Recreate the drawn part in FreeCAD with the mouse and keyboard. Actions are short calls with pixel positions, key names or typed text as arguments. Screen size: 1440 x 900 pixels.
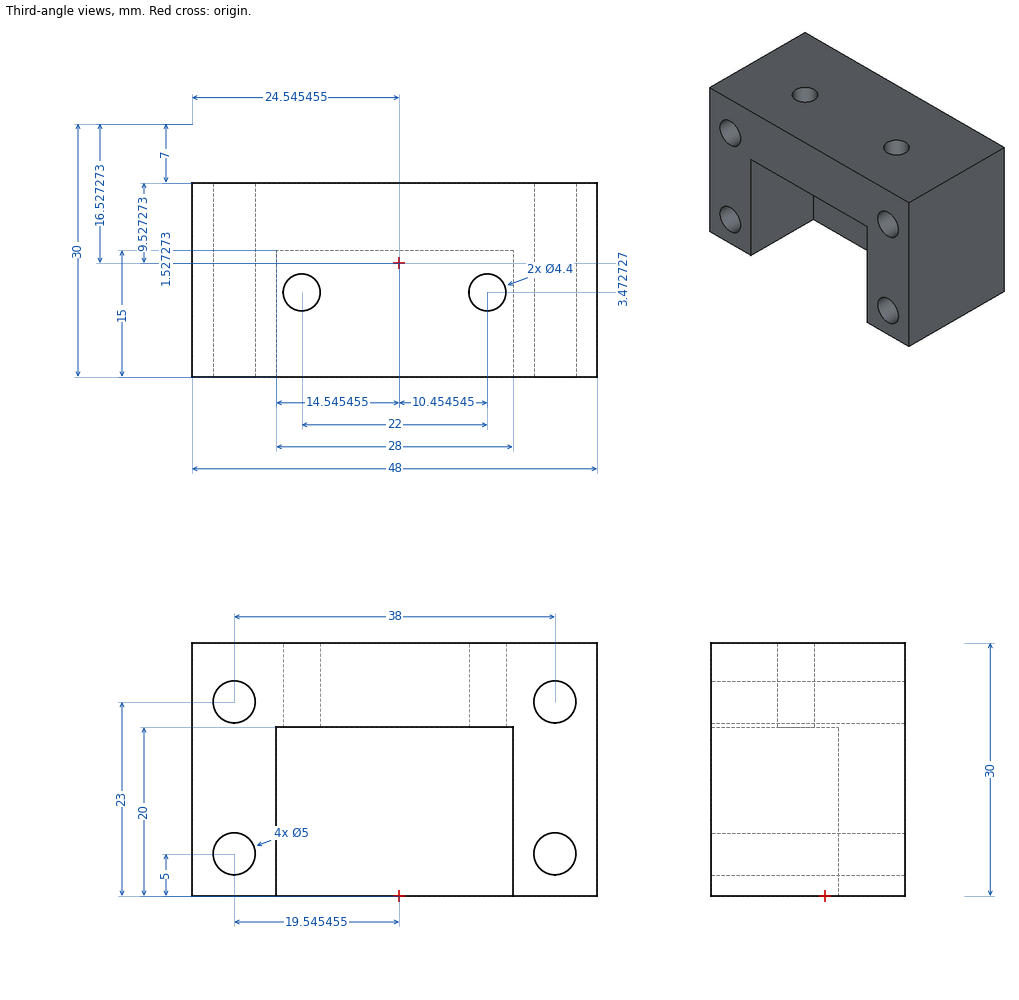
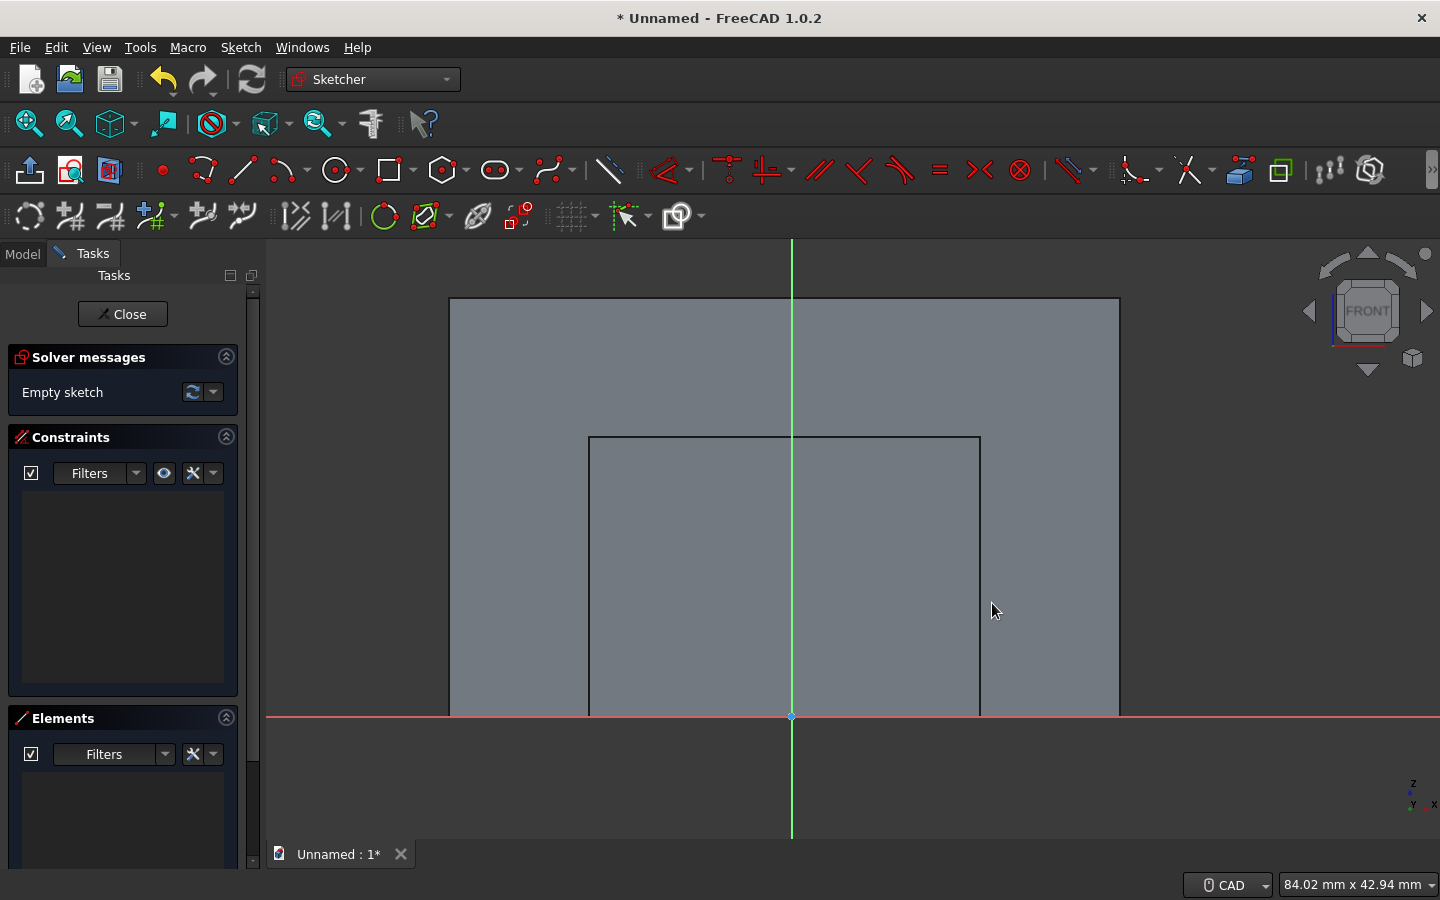
click(336, 170)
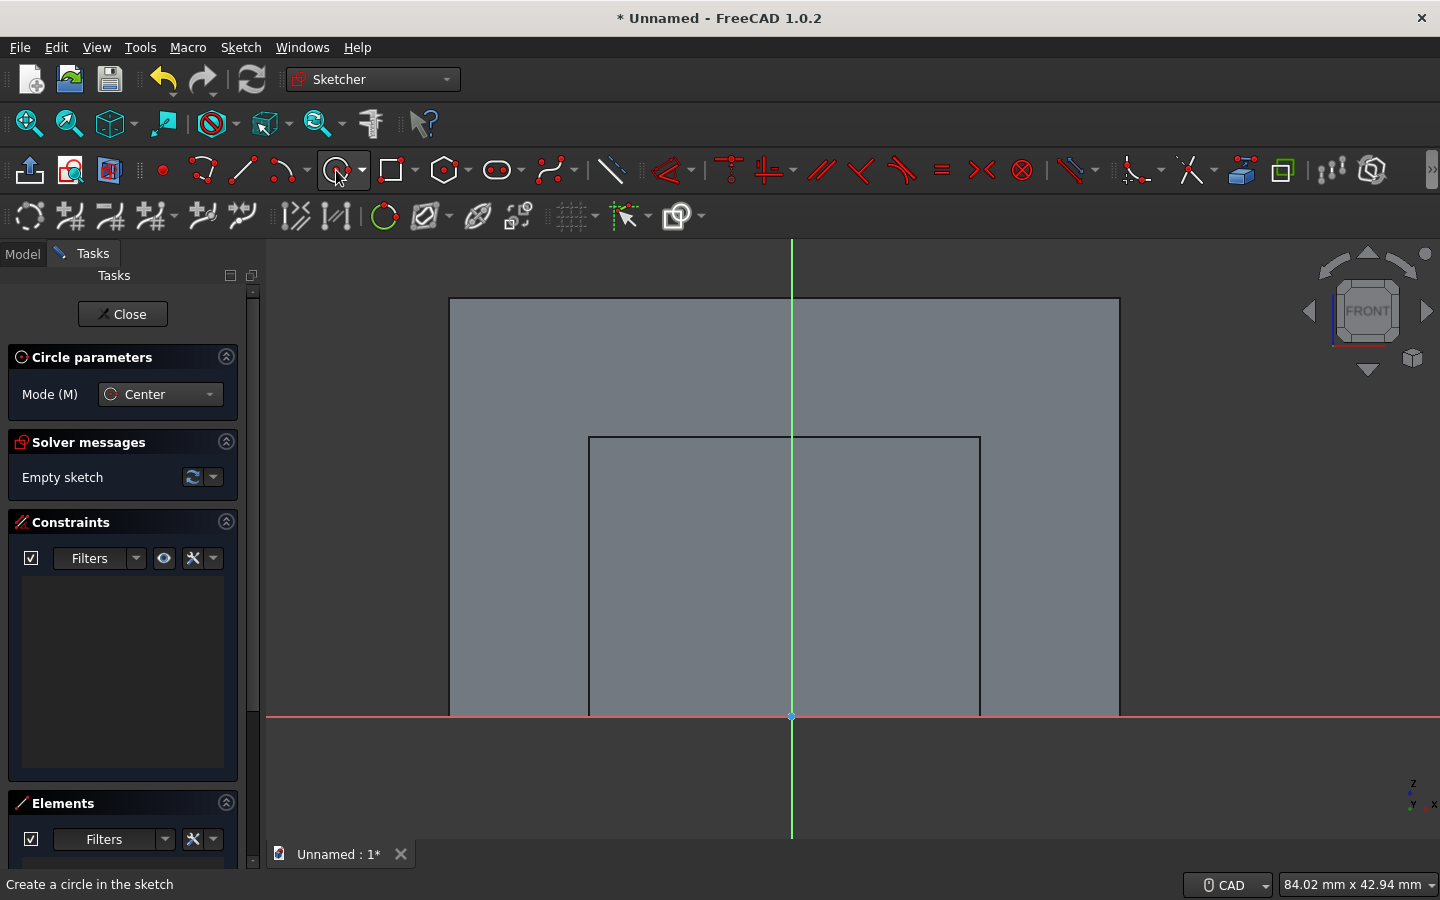
click(519, 647)
click(544, 622)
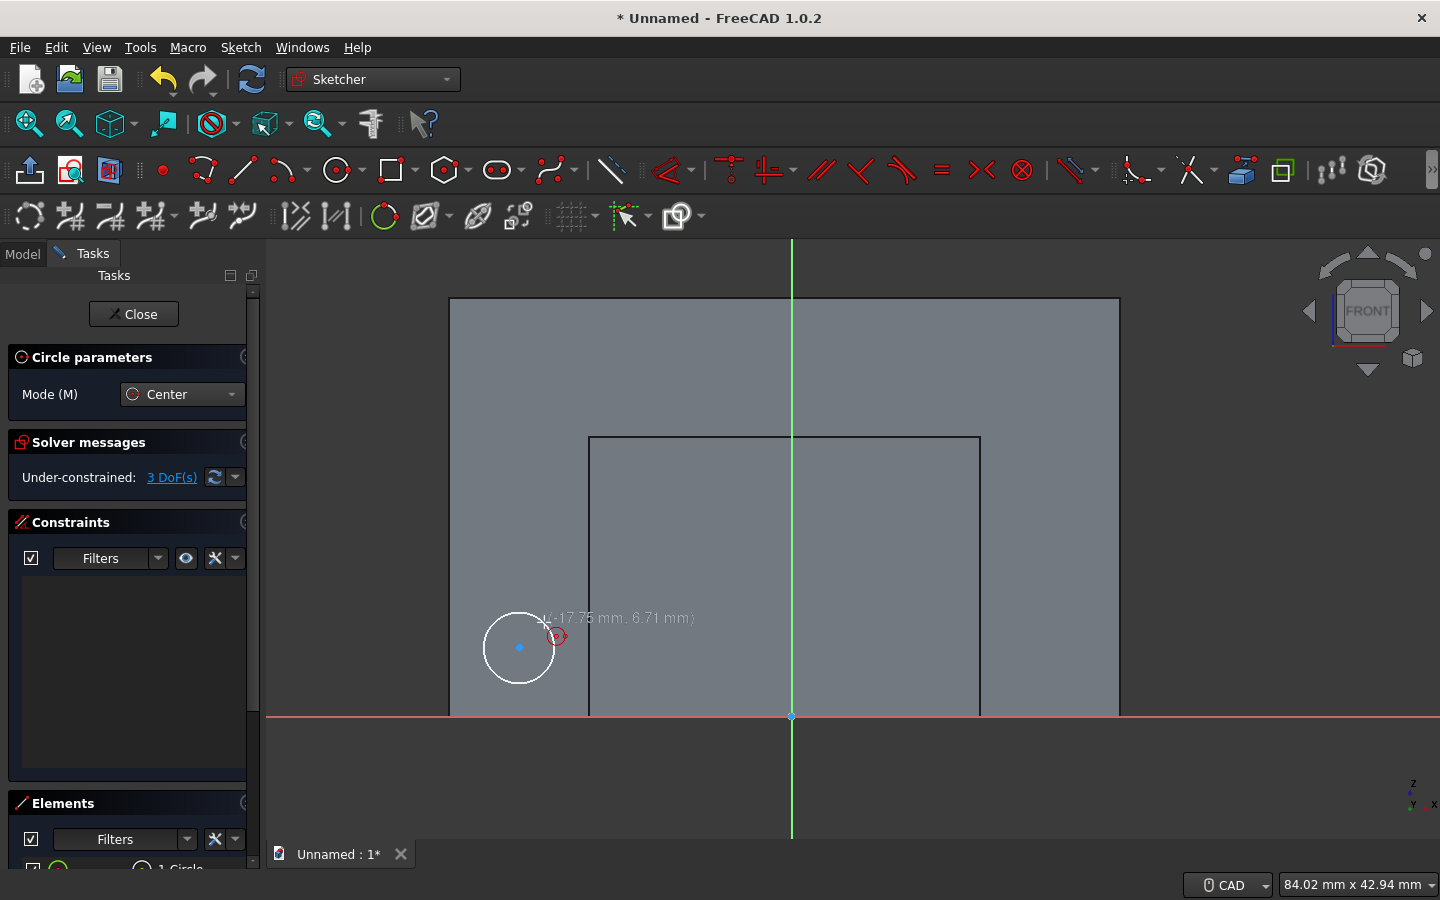
click(519, 395)
click(544, 371)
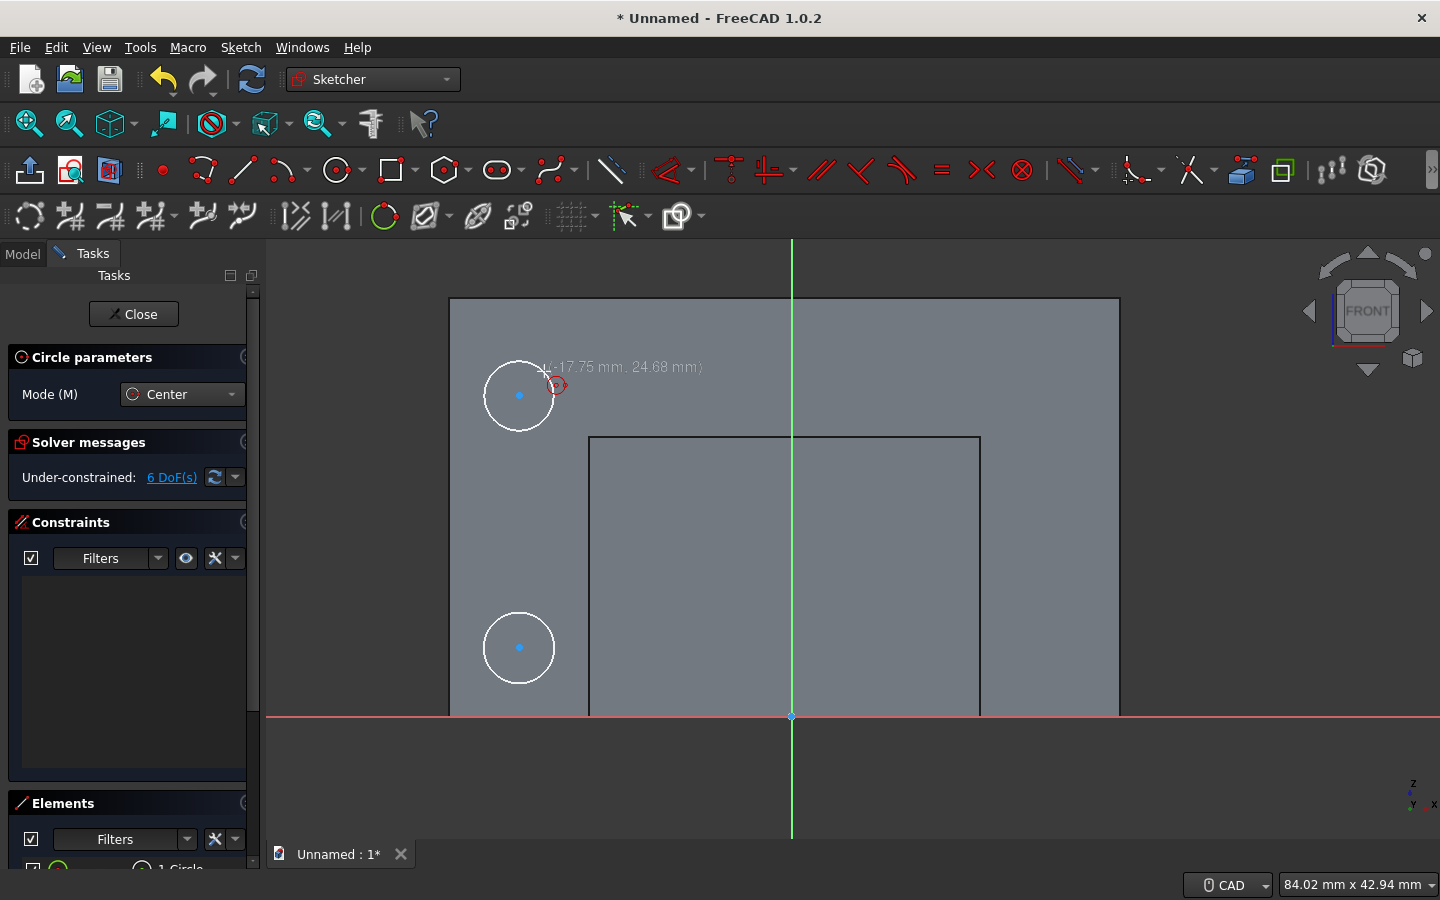
click(1050, 395)
click(1075, 371)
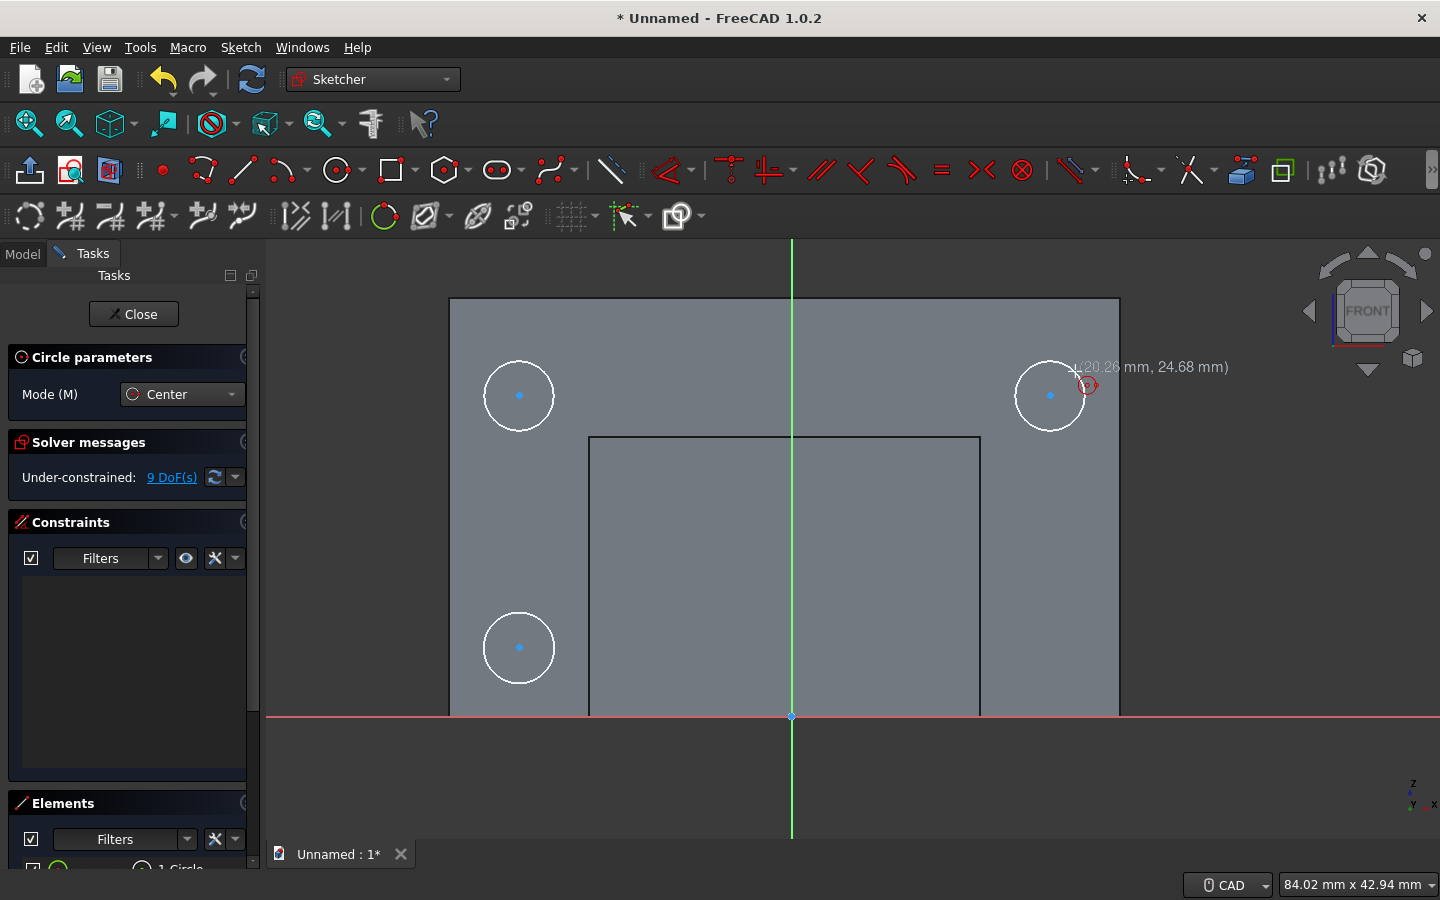
click(1050, 647)
click(1075, 622)
key(Escape)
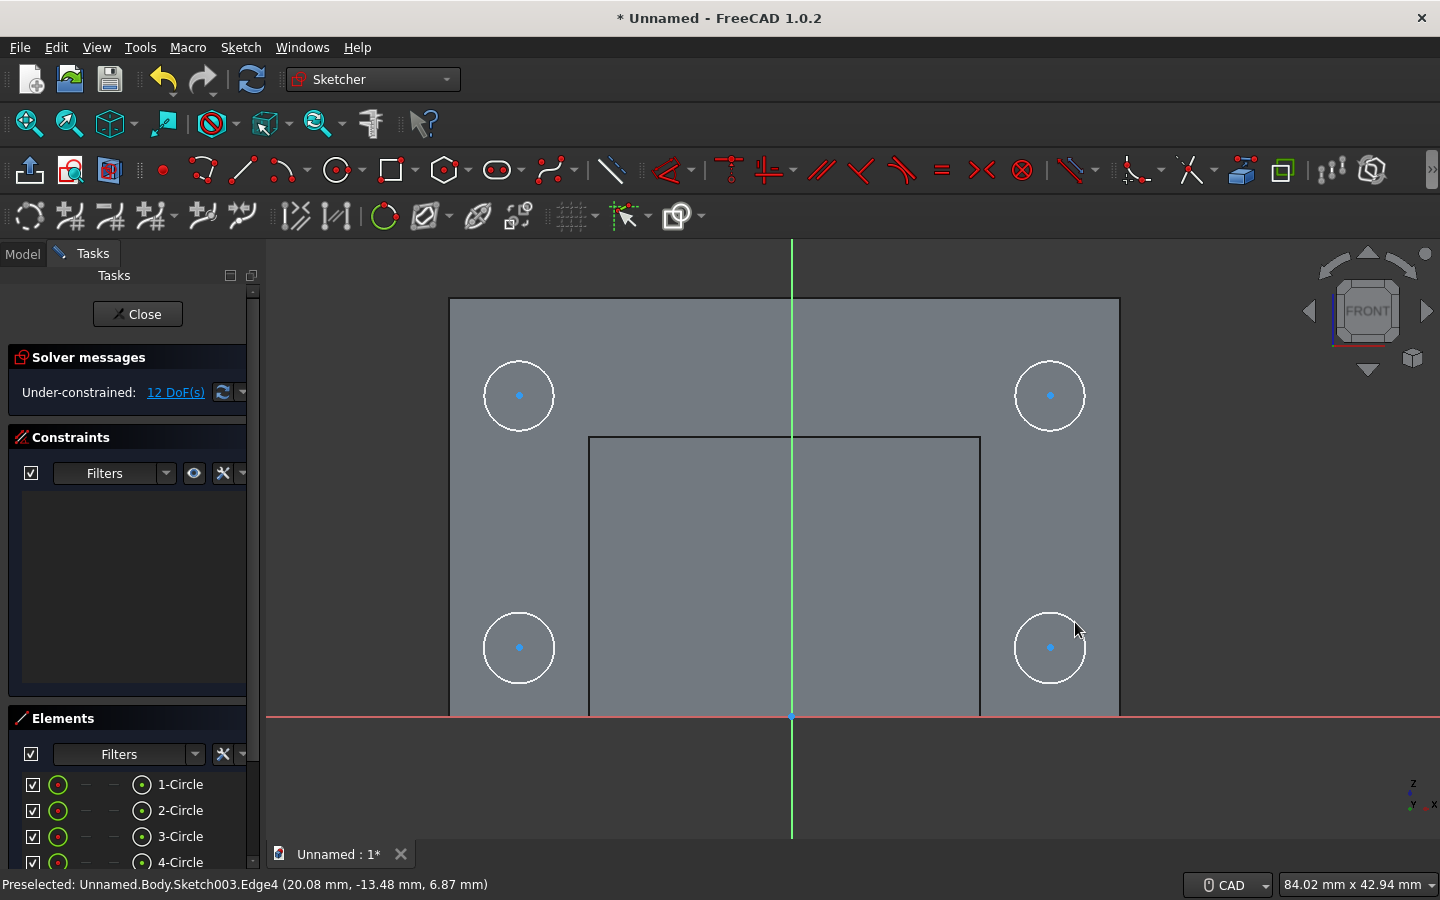
click(544, 623)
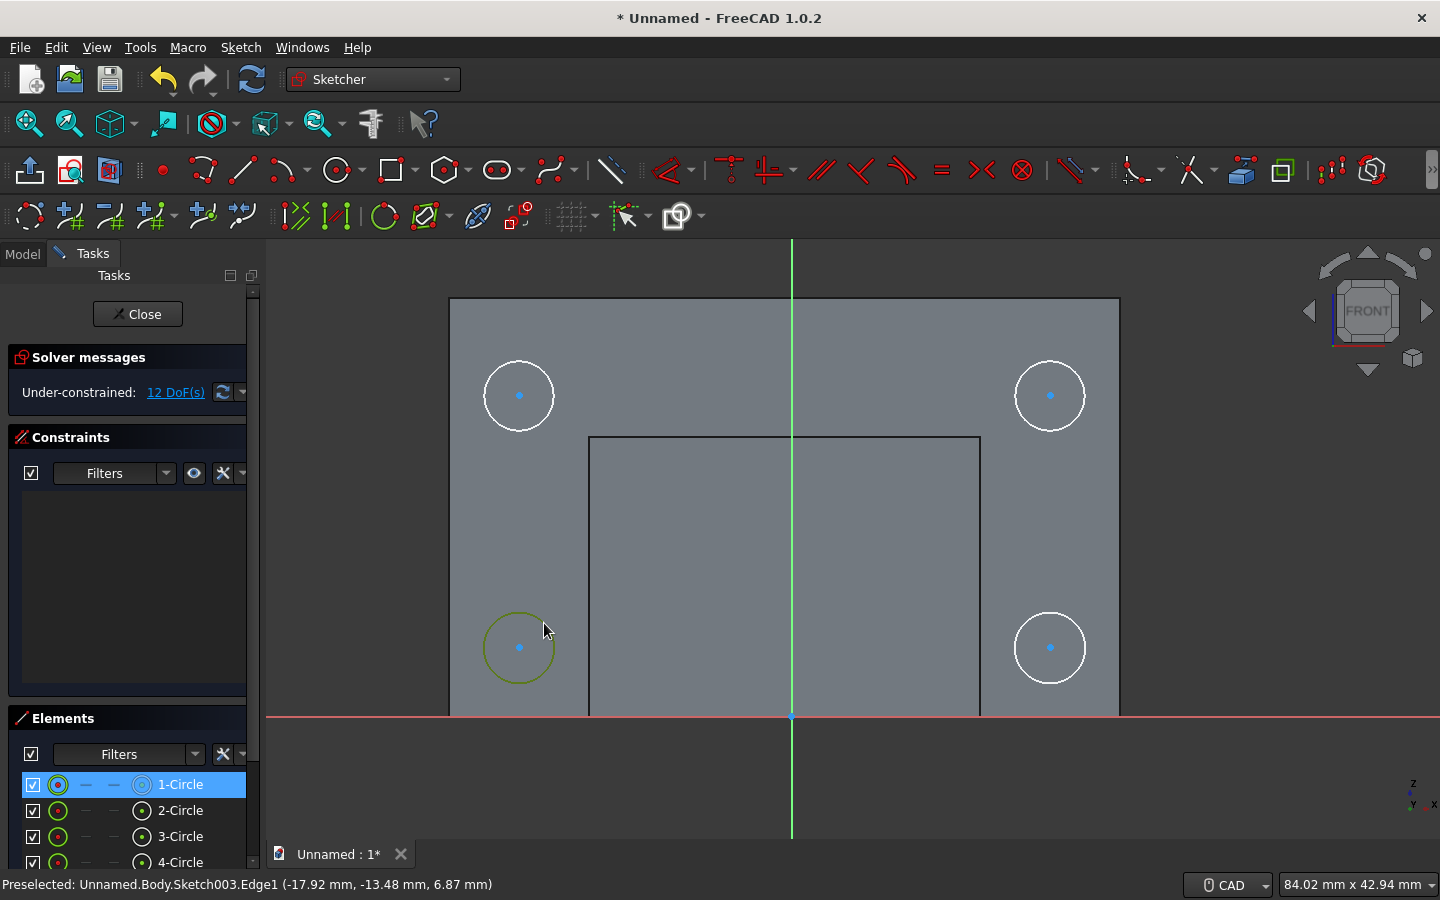
click(543, 371)